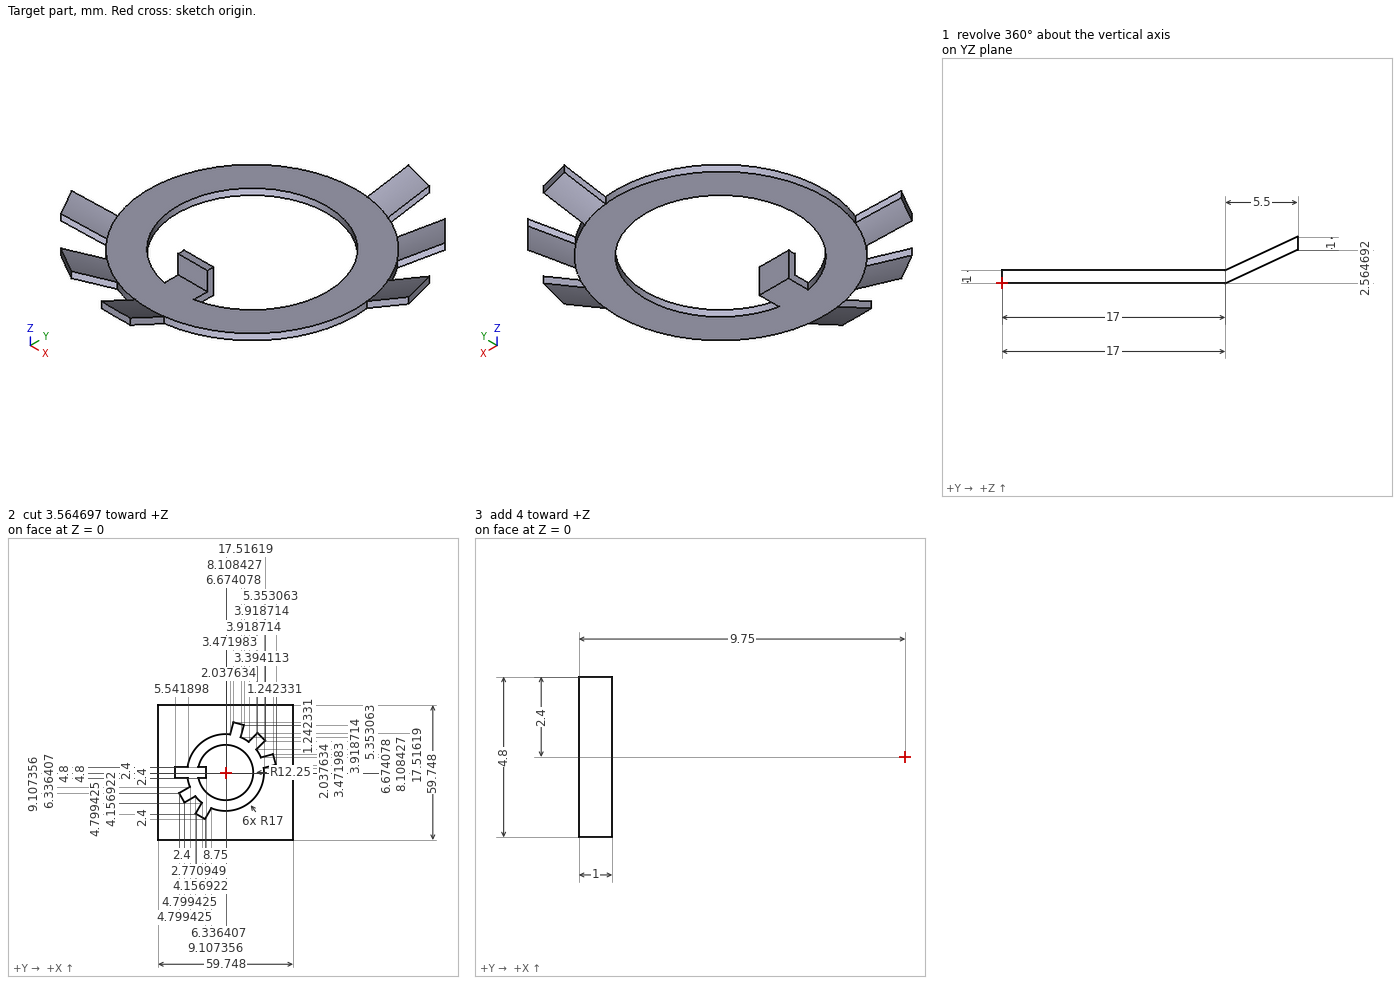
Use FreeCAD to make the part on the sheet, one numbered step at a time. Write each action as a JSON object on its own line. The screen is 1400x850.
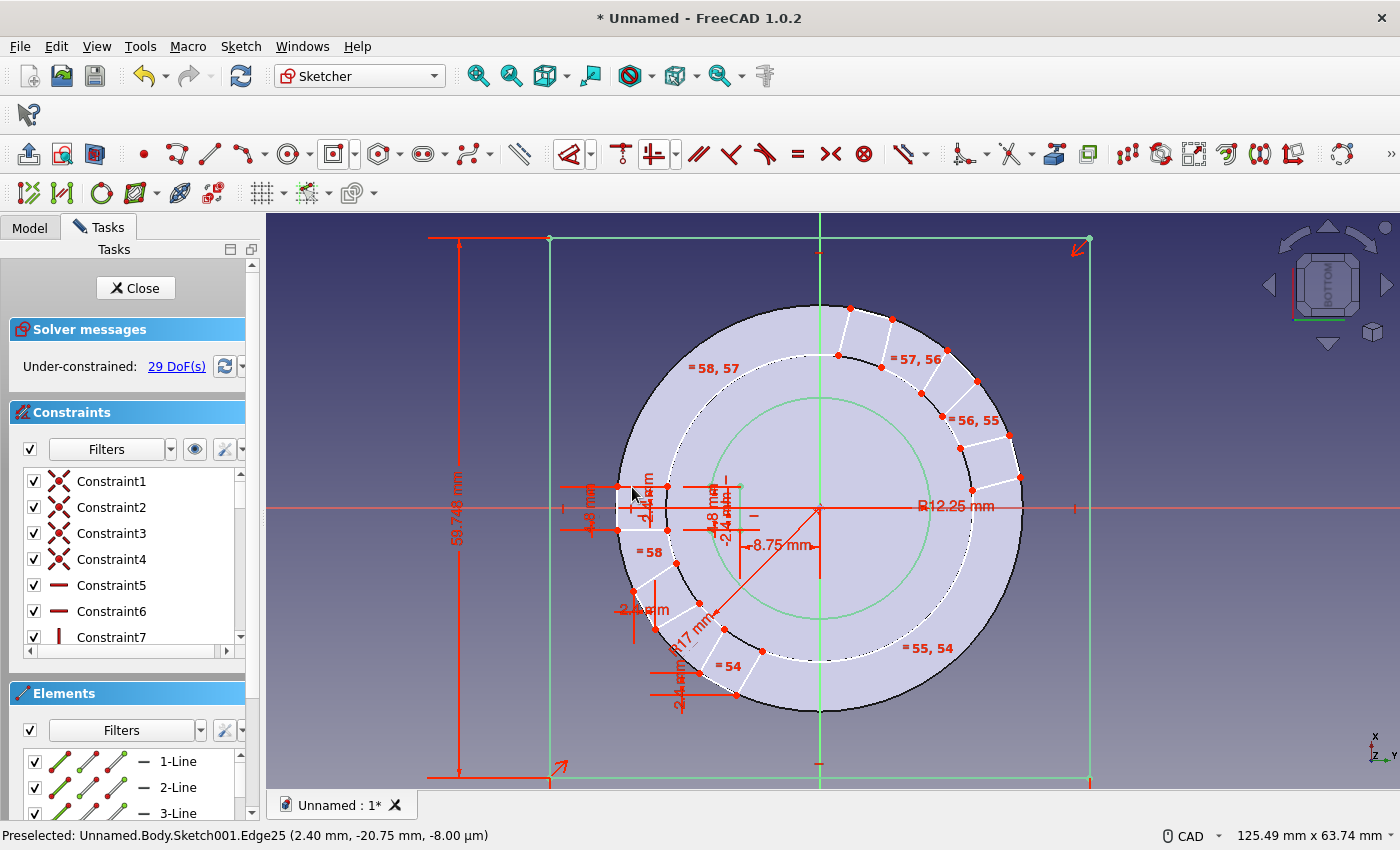
{"action": "key", "text": "l"}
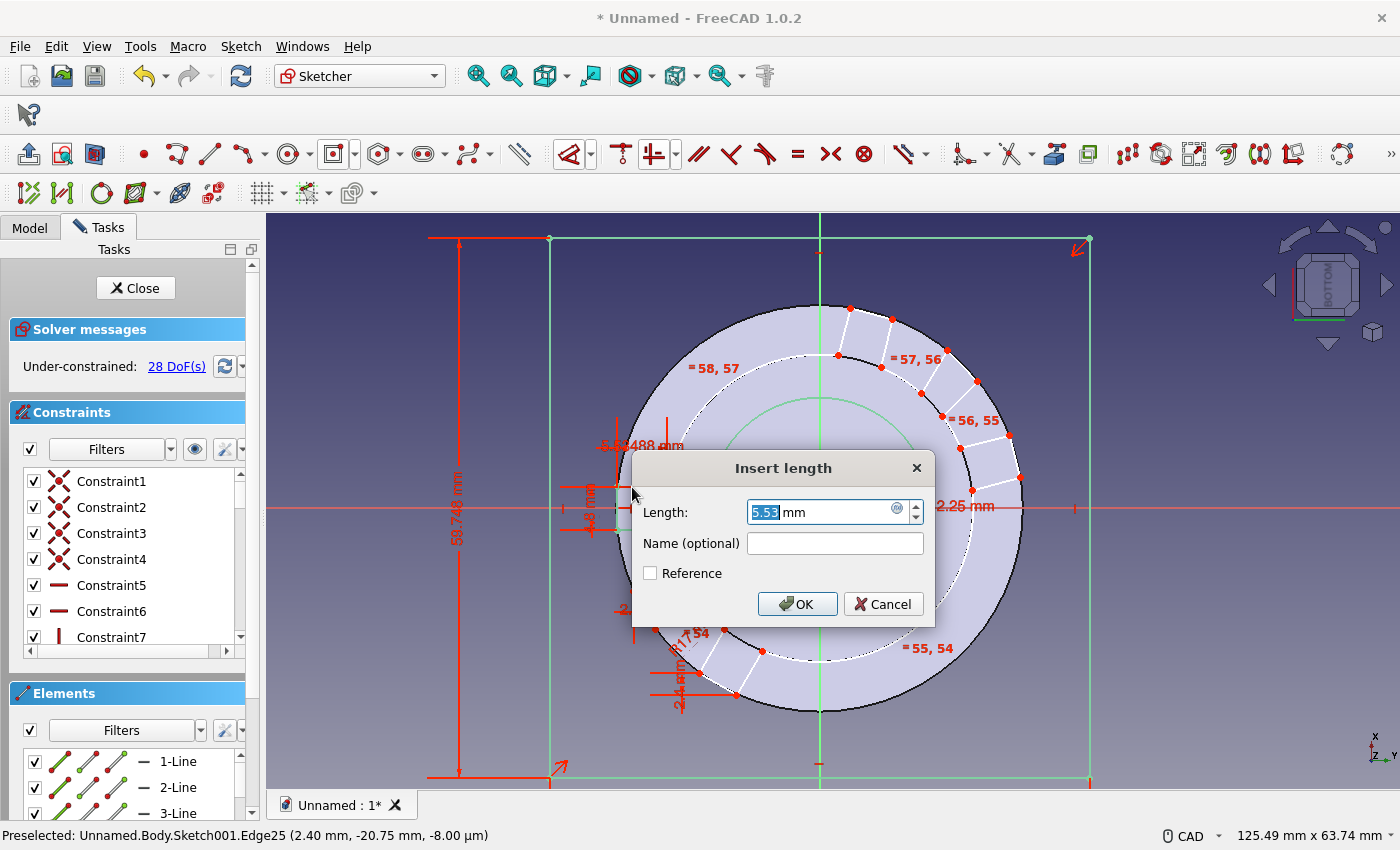
{"action": "type", "text": "5.541898"}
{"action": "key", "text": "Return"}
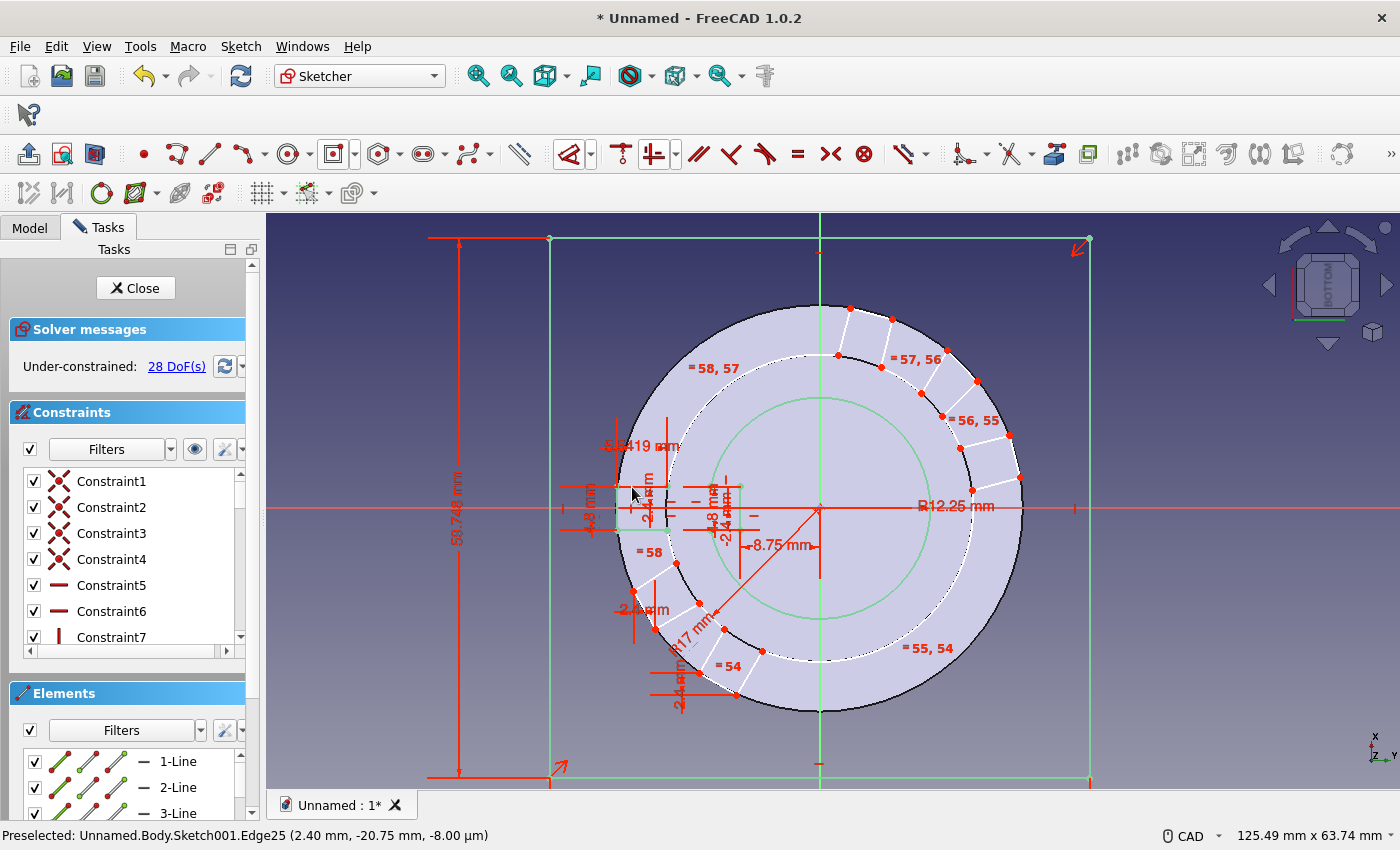
{"action": "left_click", "coordinate": [676, 563]}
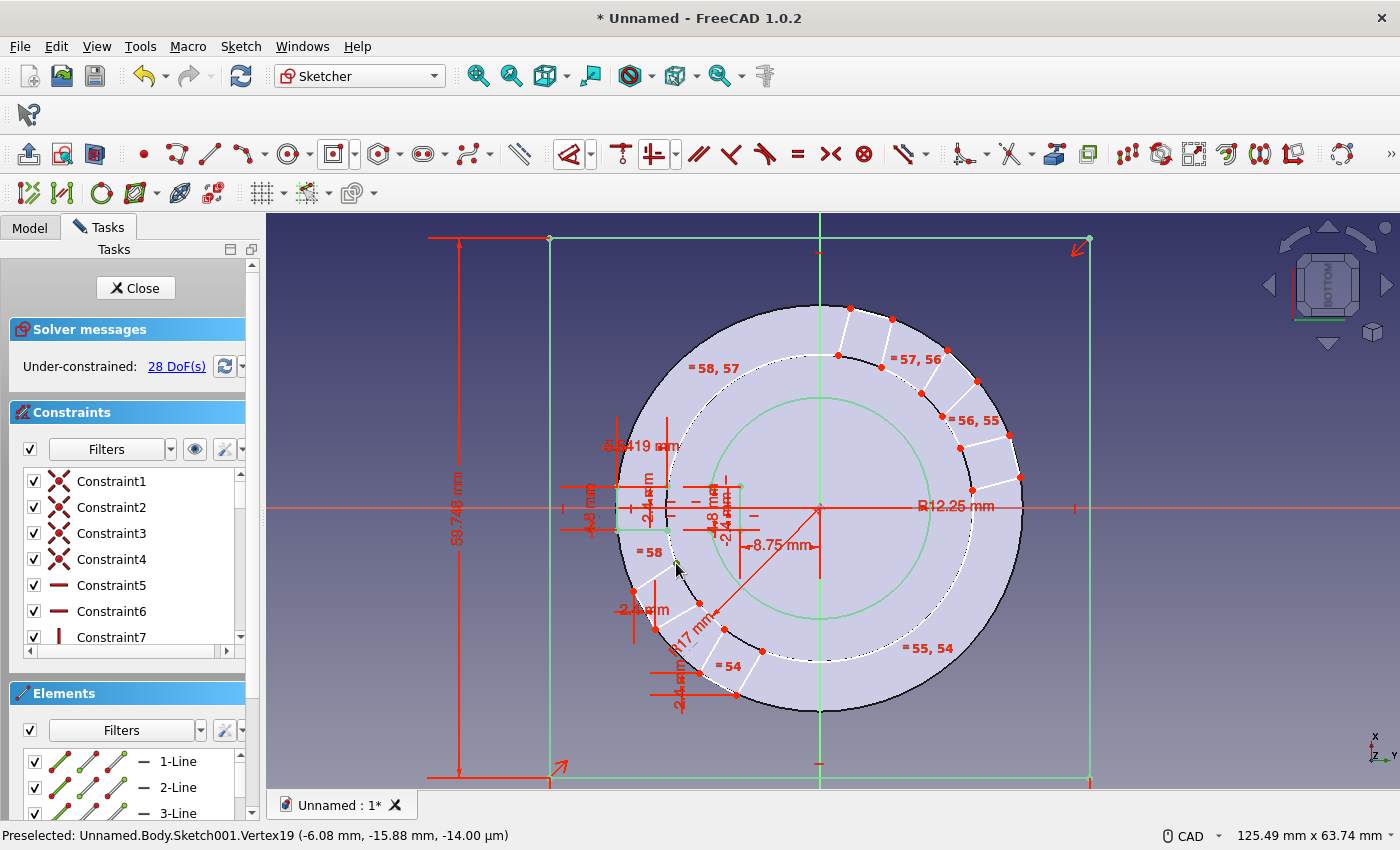
{"action": "key", "text": "i"}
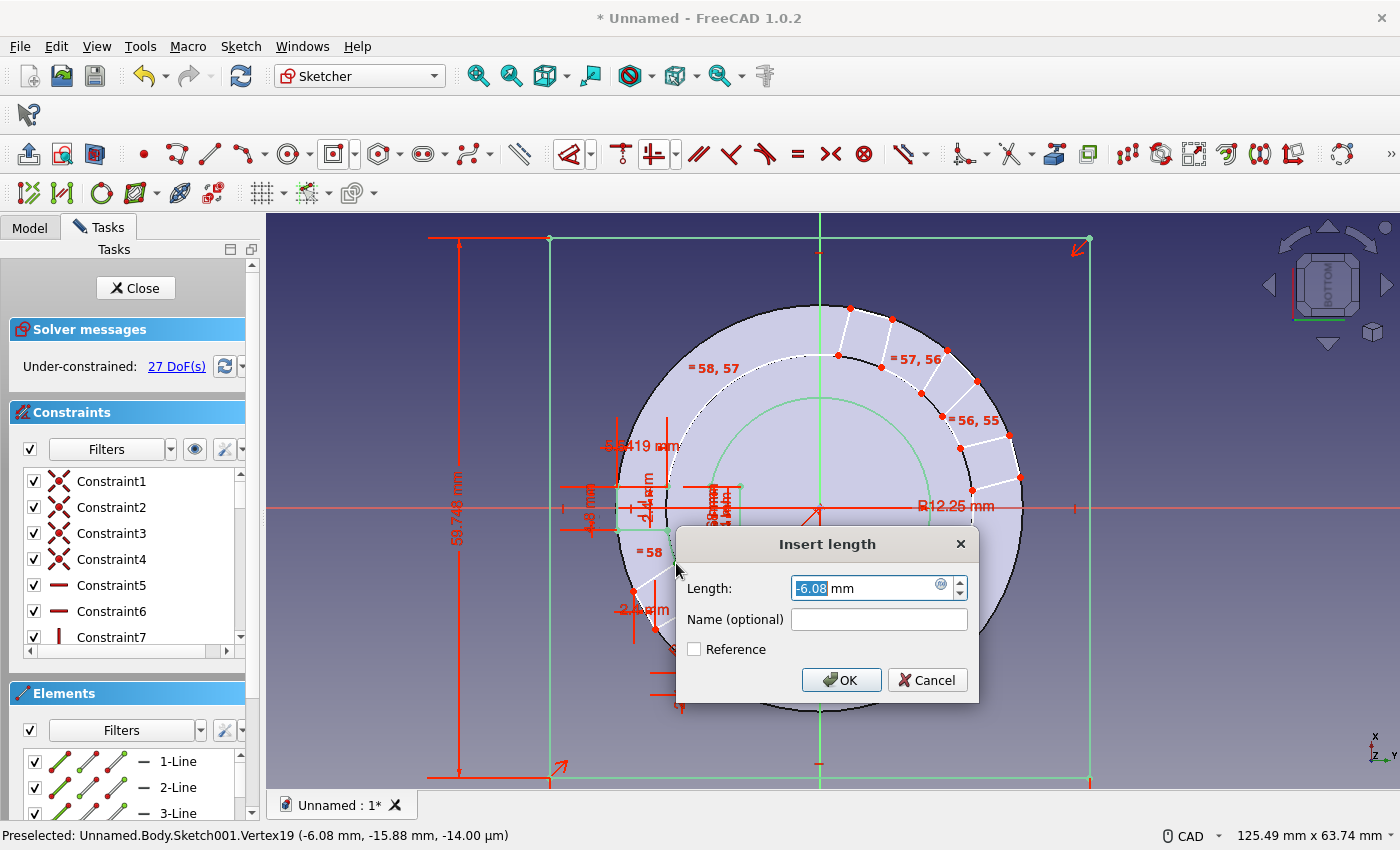
{"action": "type", "text": "-6.336407"}
{"action": "key", "text": "Return"}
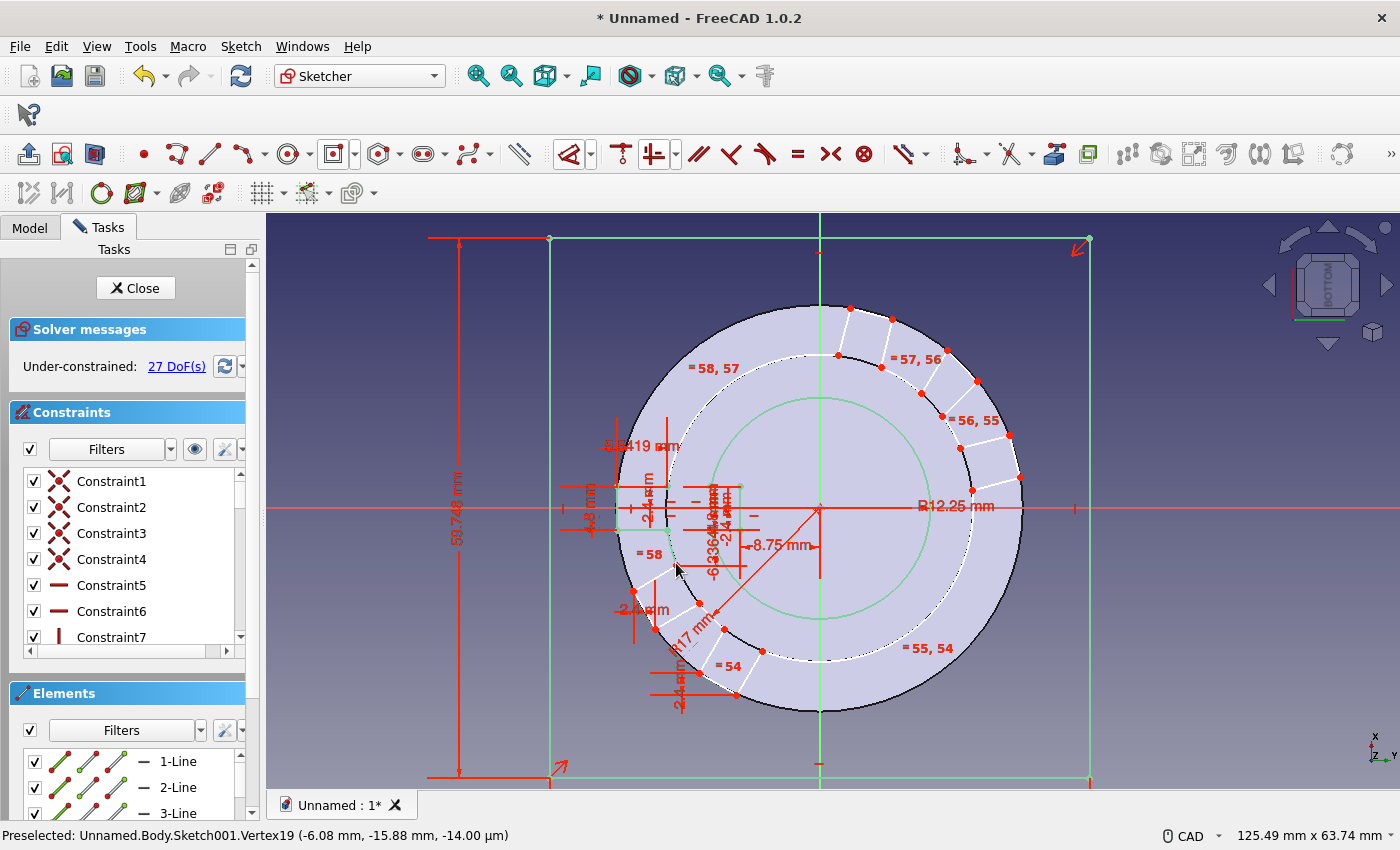
{"action": "left_click", "coordinate": [634, 591]}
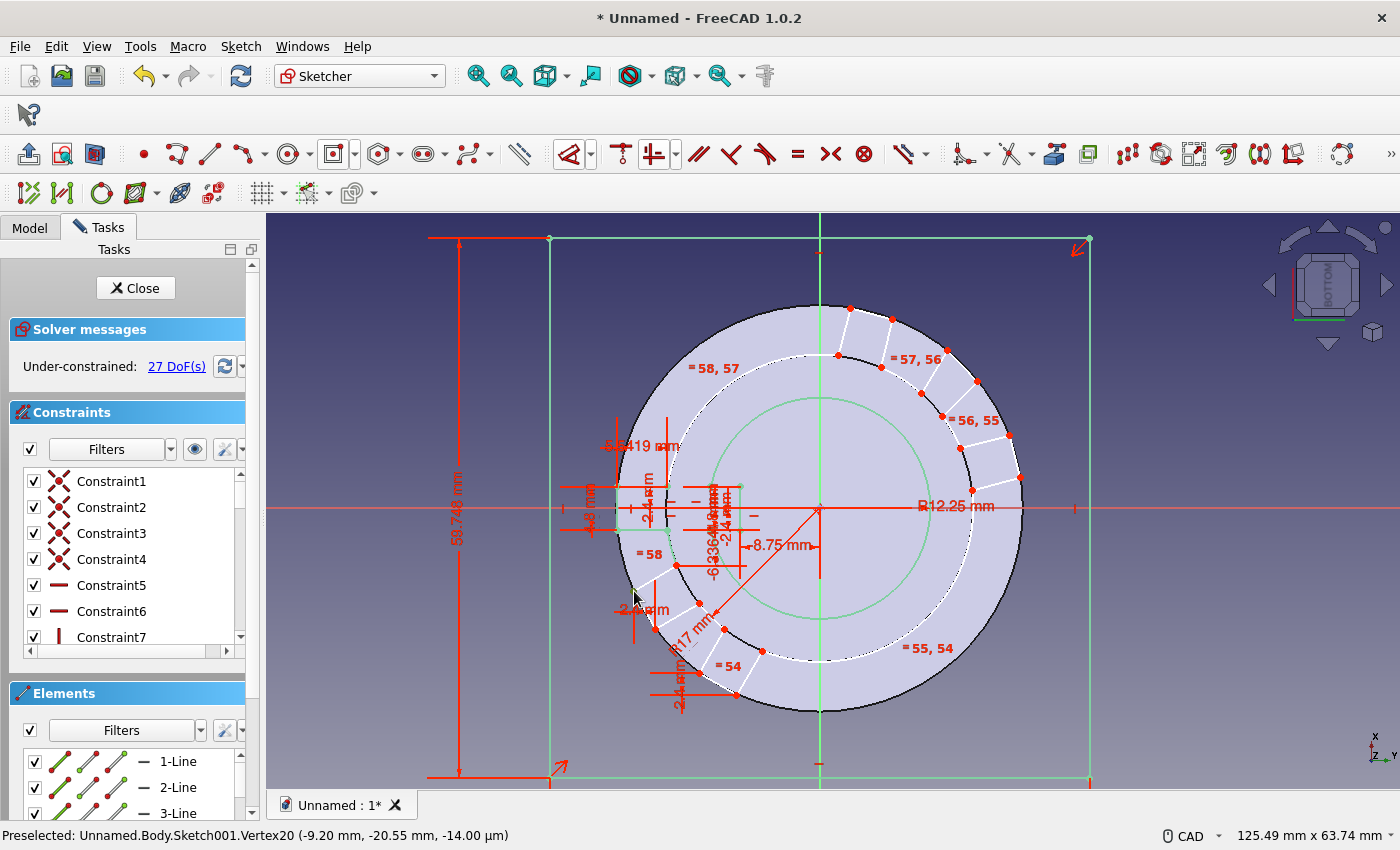
{"action": "left_click", "coordinate": [590, 154]}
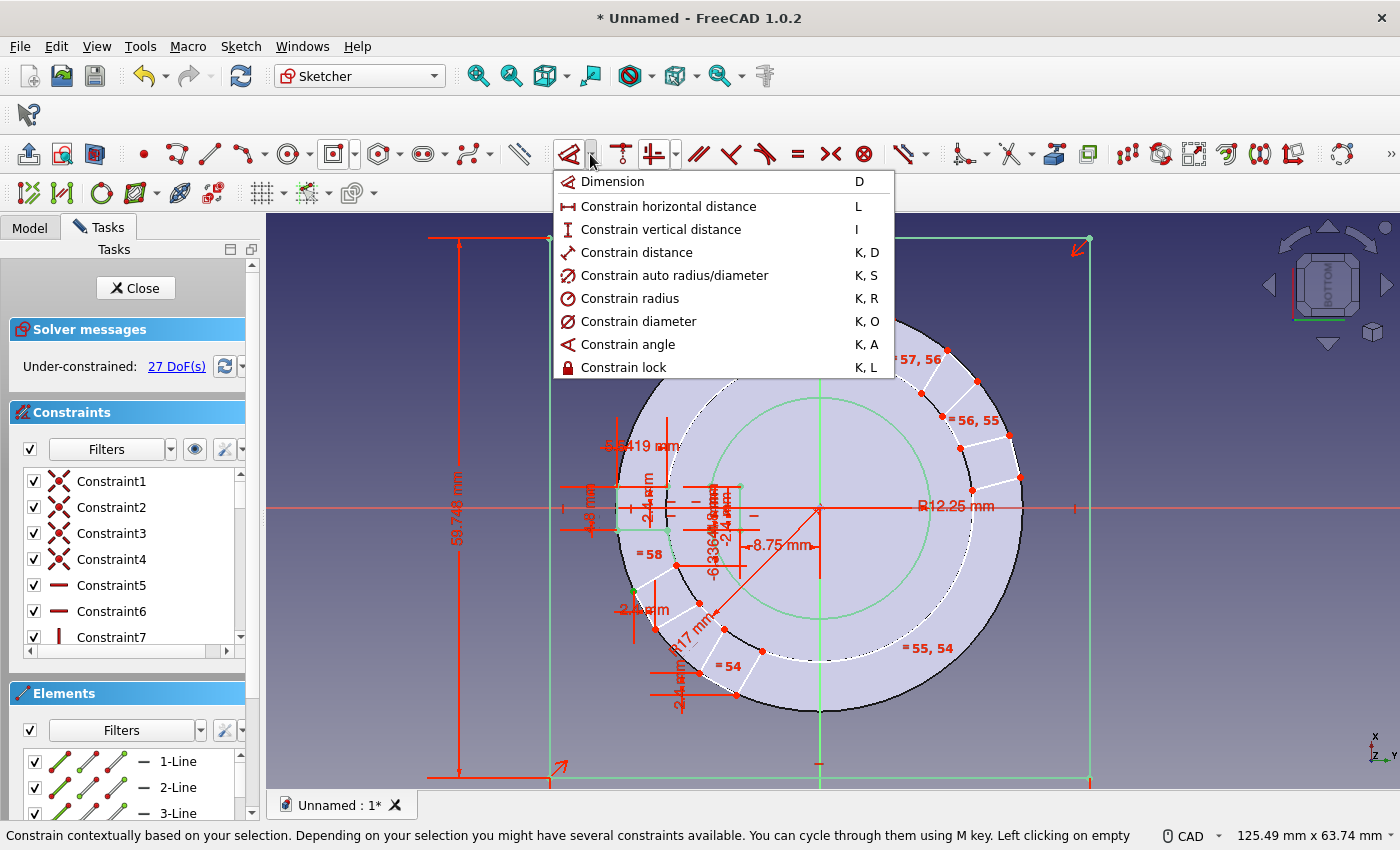
{"action": "left_click", "coordinate": [724, 230]}